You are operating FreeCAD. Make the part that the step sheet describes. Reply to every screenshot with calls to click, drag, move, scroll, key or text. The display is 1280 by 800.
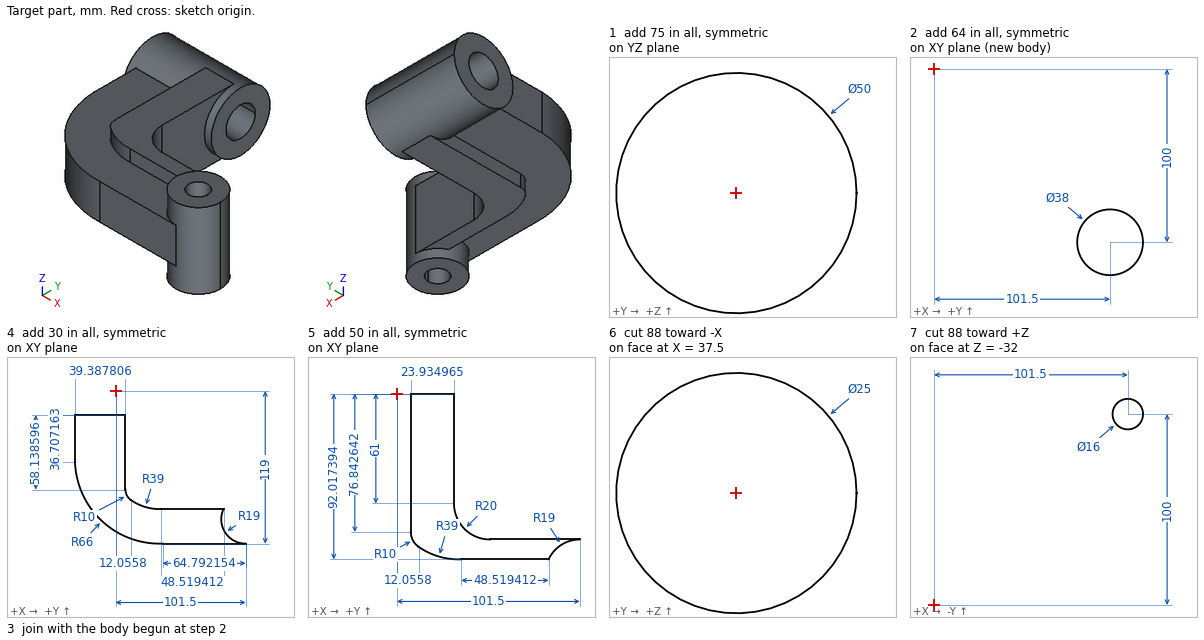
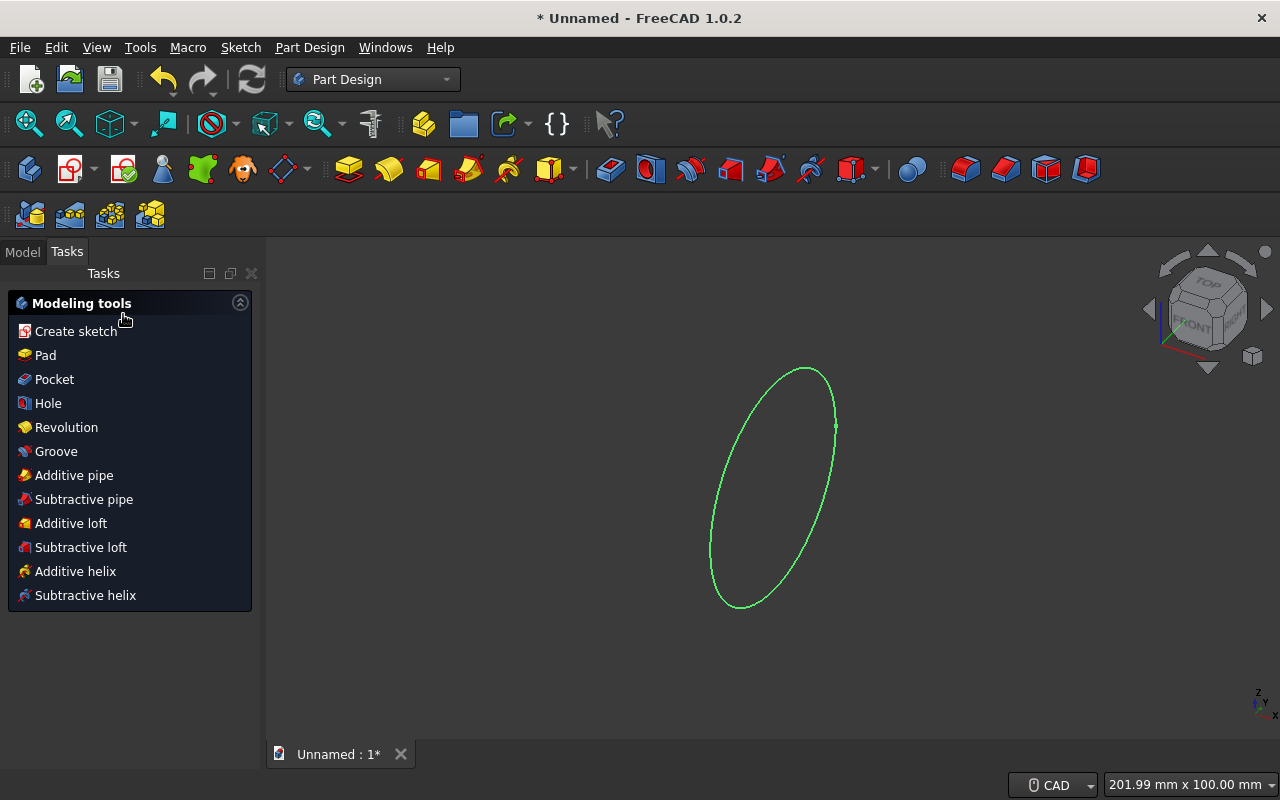
click(350, 170)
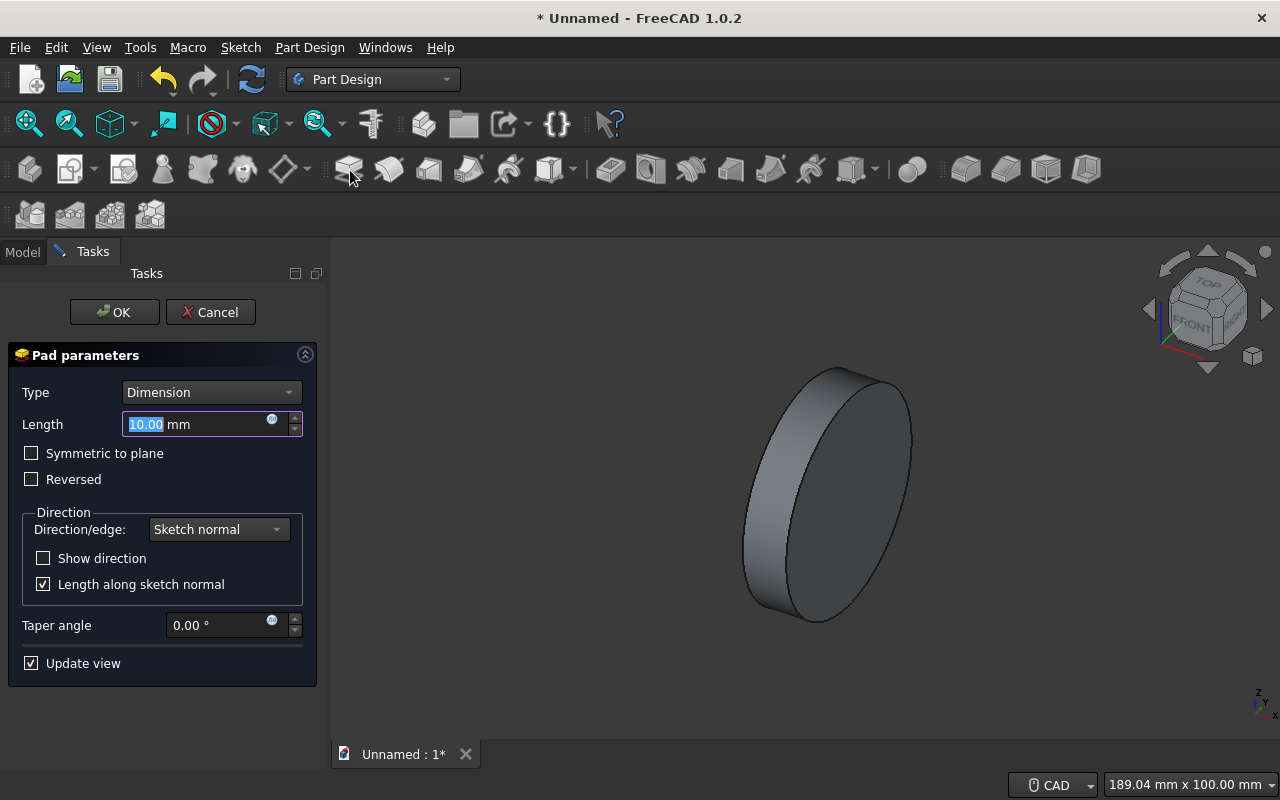
text(75)
key(Tab)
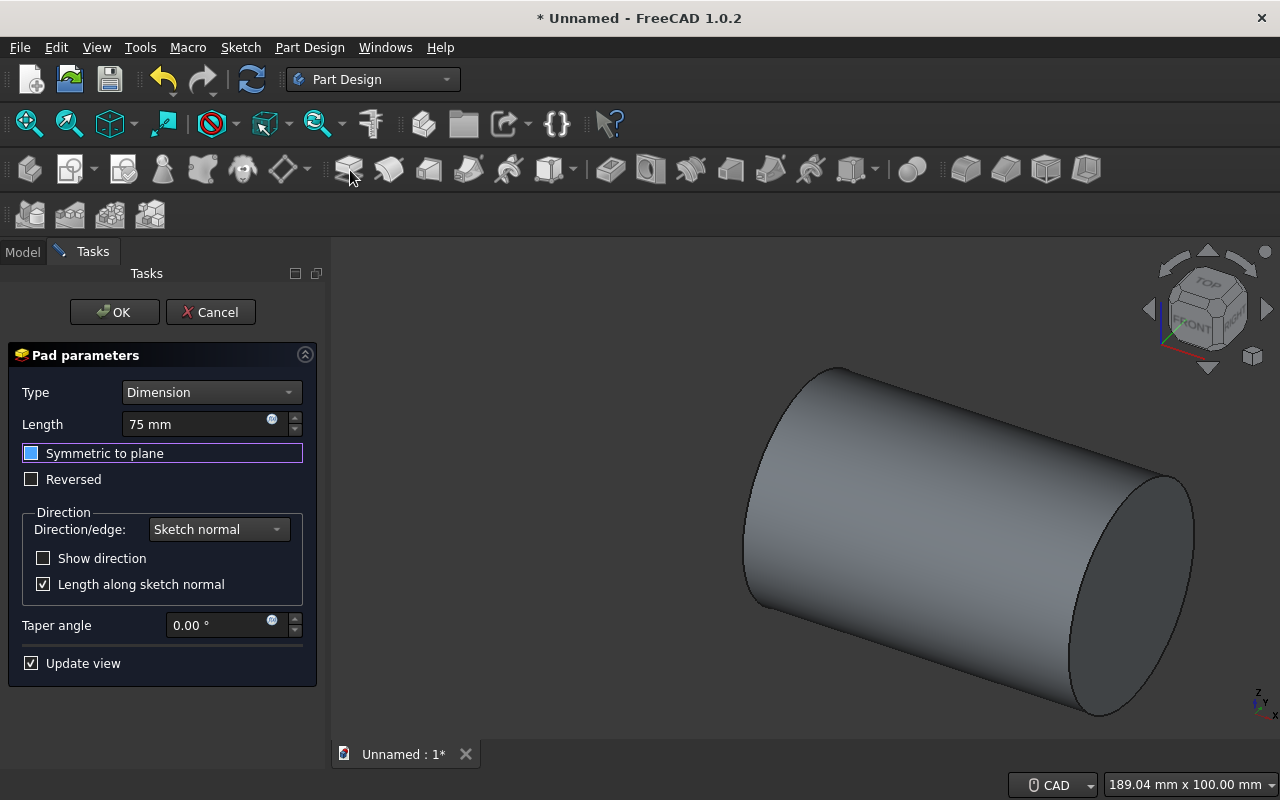
click(30, 453)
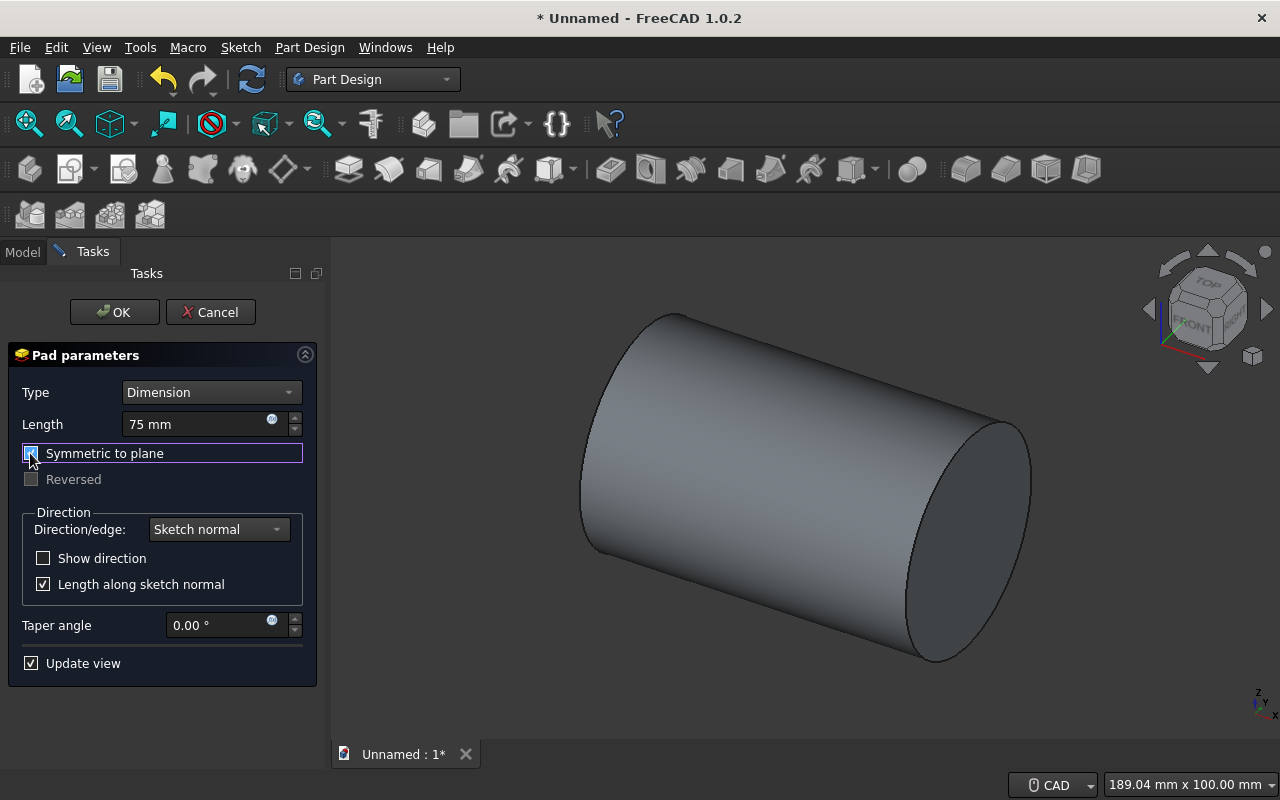
click(115, 312)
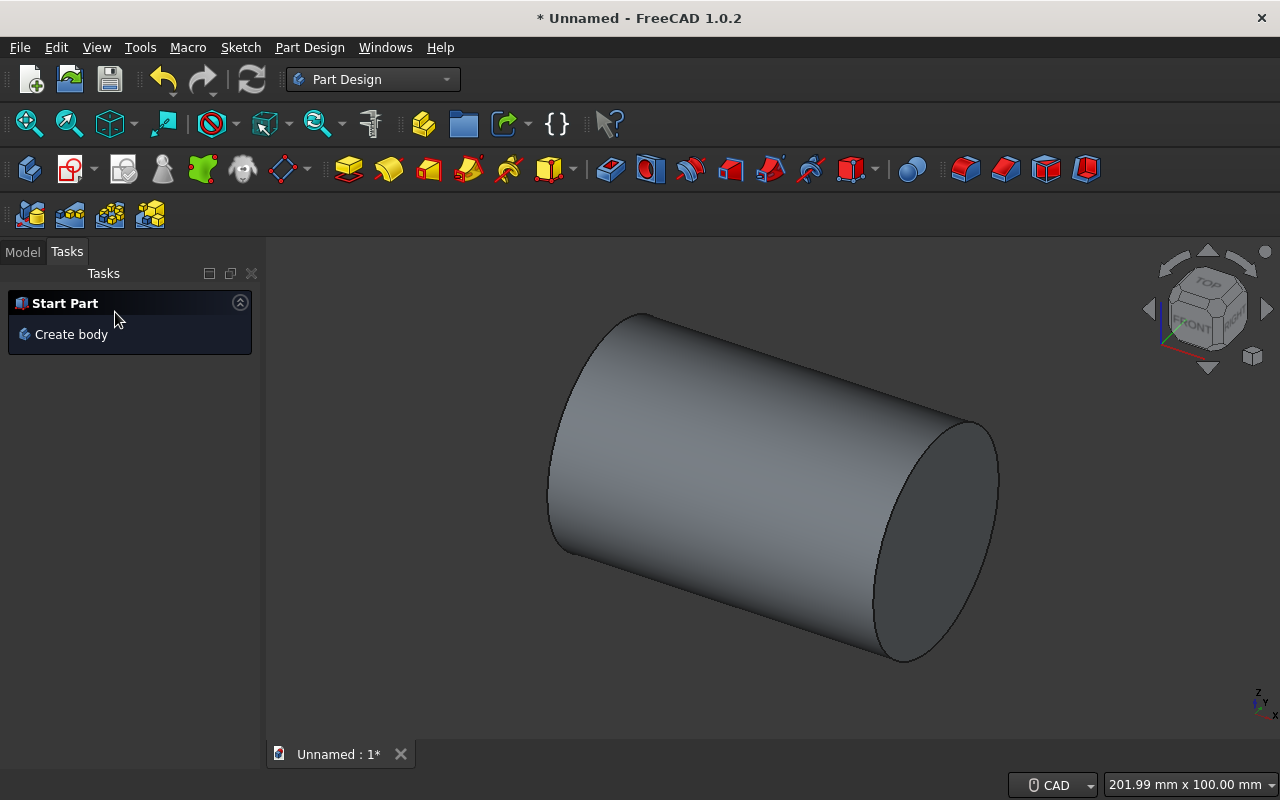
click(30, 170)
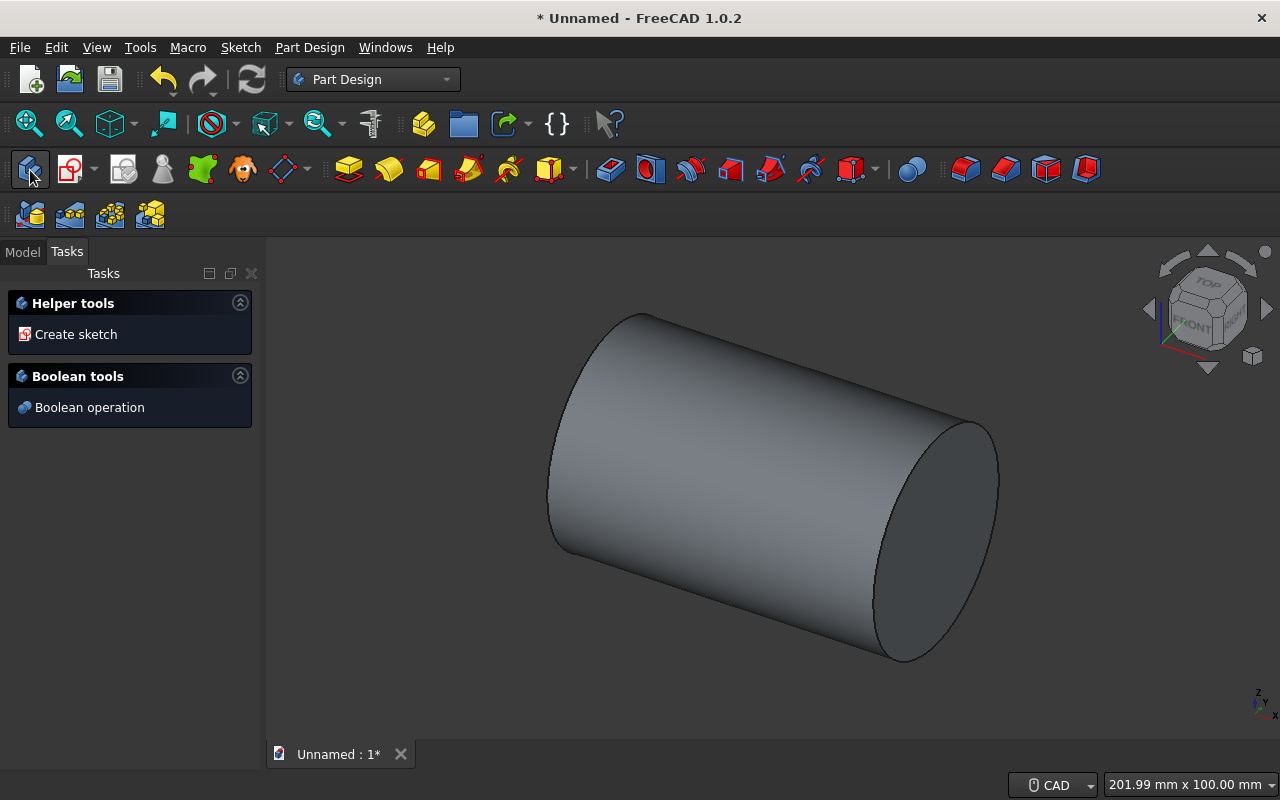
click(306, 699)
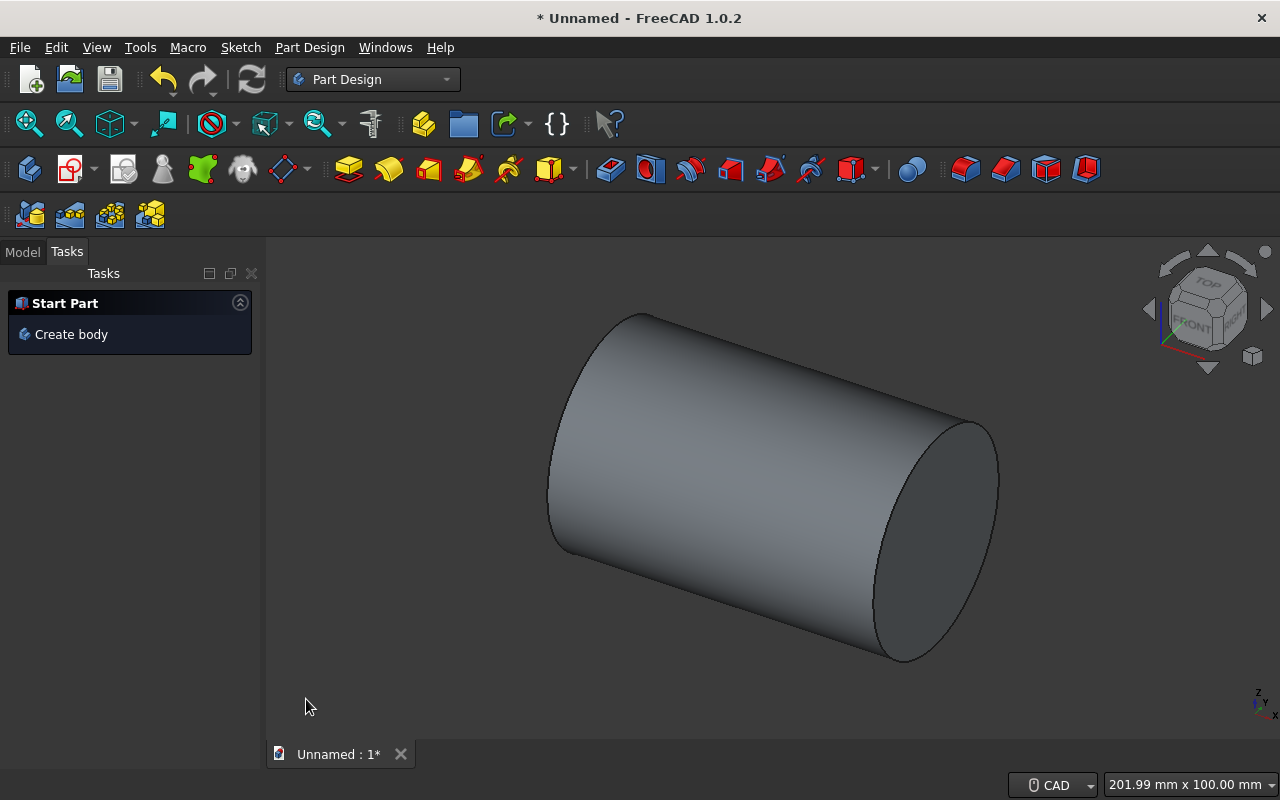
click(70, 170)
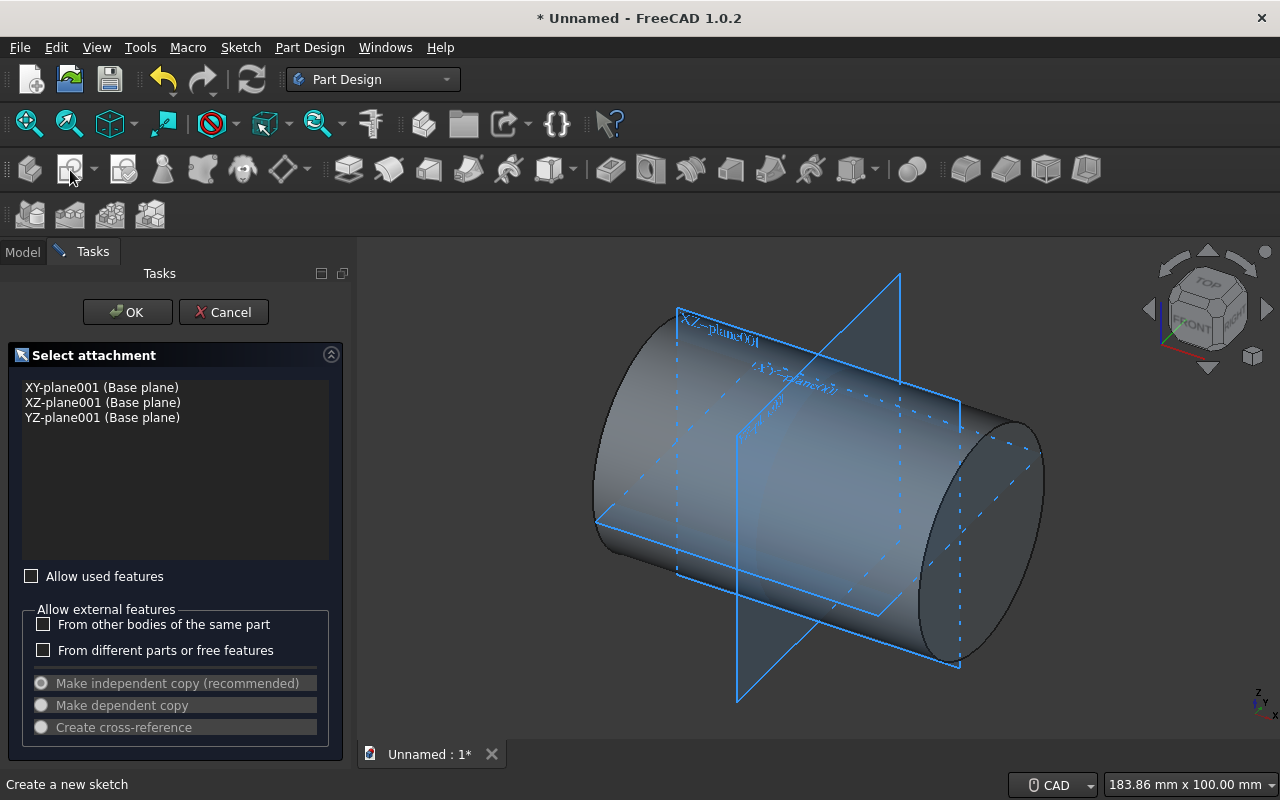
click(82, 388)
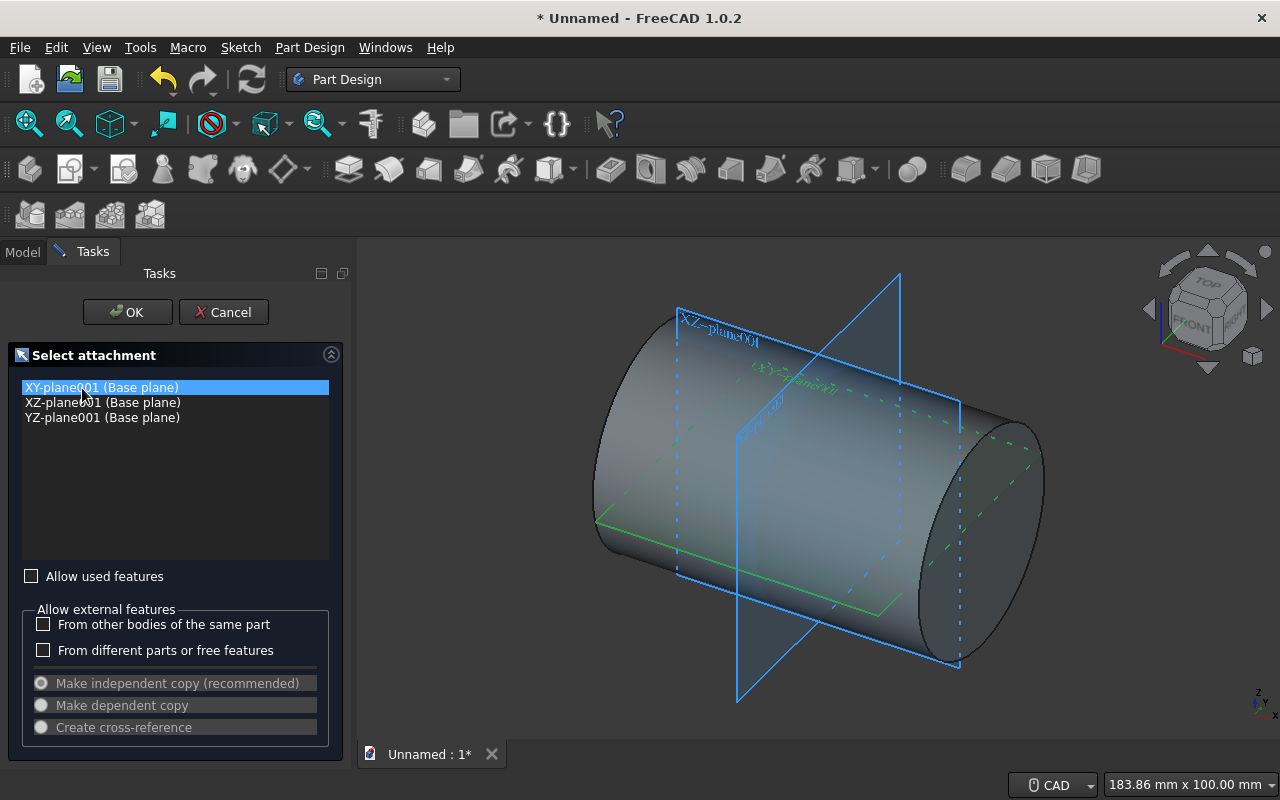
click(128, 312)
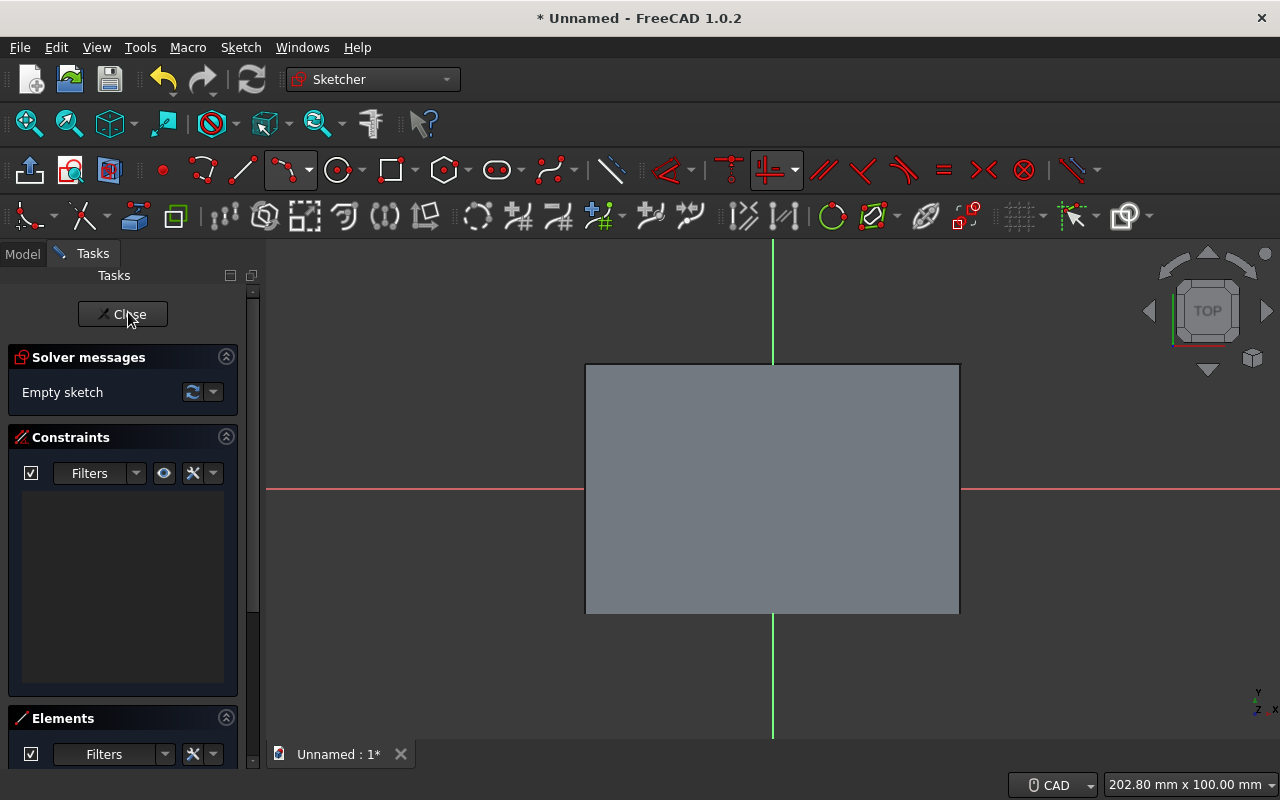
scroll(704, 489, down, 5)